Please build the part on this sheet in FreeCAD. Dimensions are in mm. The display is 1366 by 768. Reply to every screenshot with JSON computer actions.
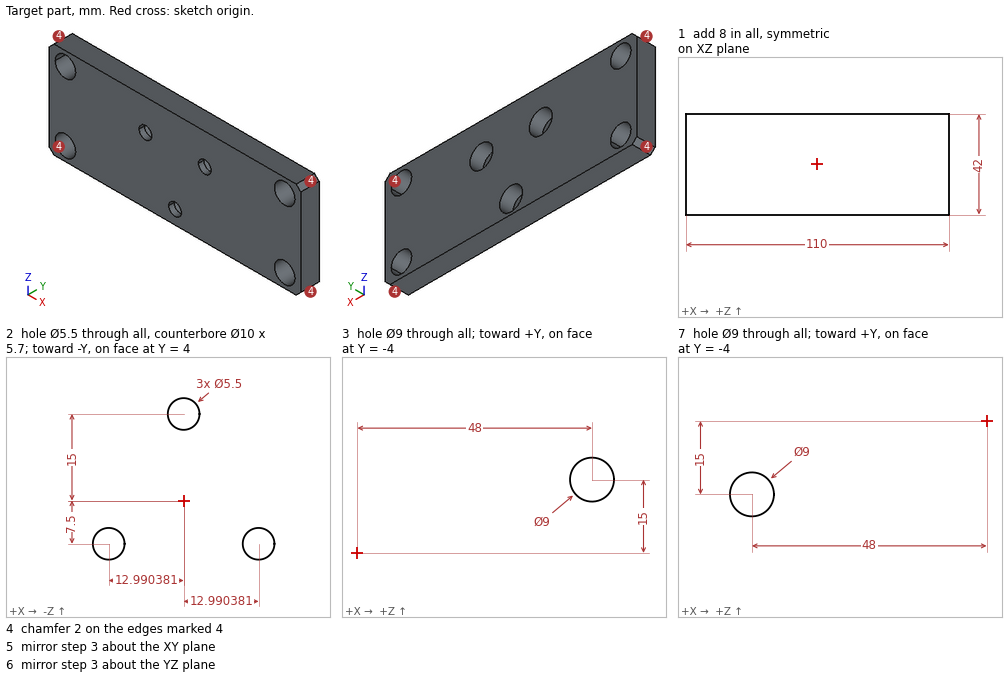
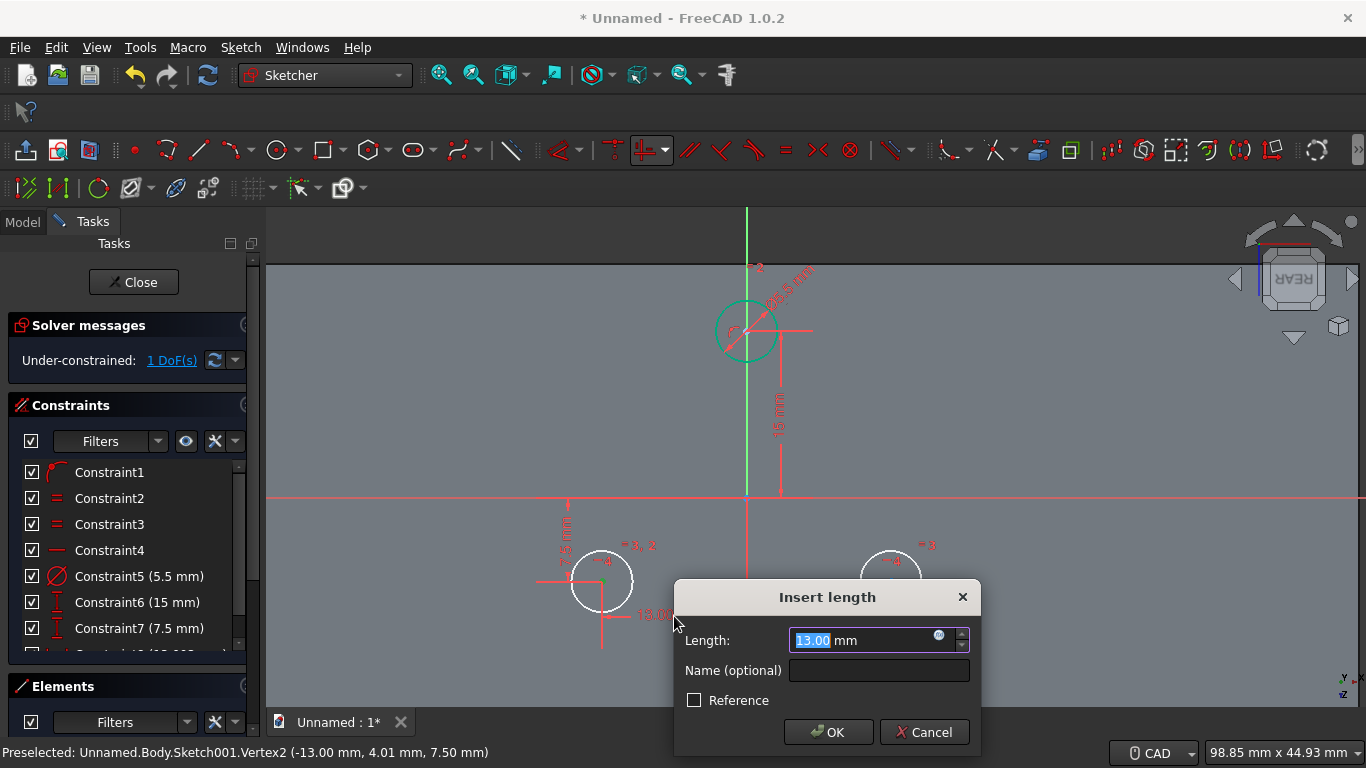
{"action": "type", "text": "12.990381"}
{"action": "key", "text": "Return"}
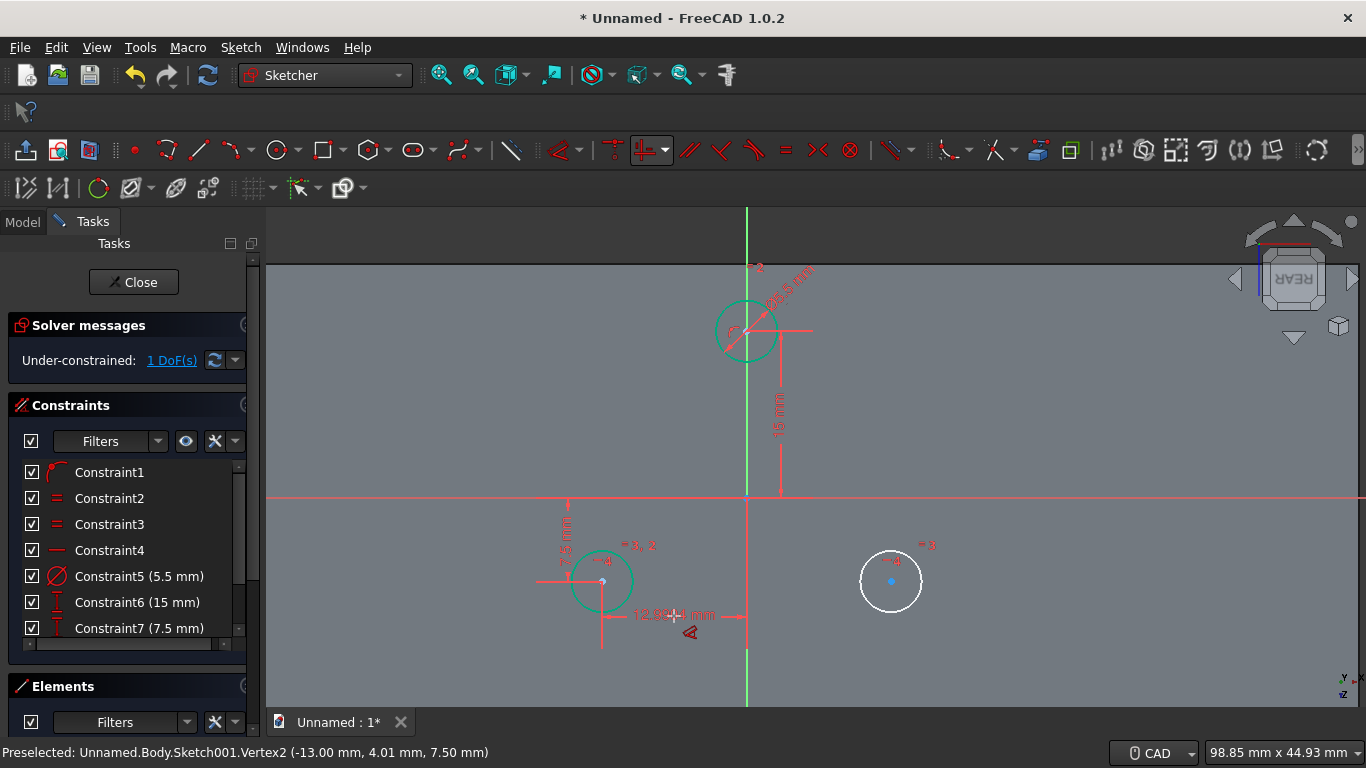
{"action": "left_click", "coordinate": [891, 582]}
{"action": "left_click", "coordinate": [819, 616]}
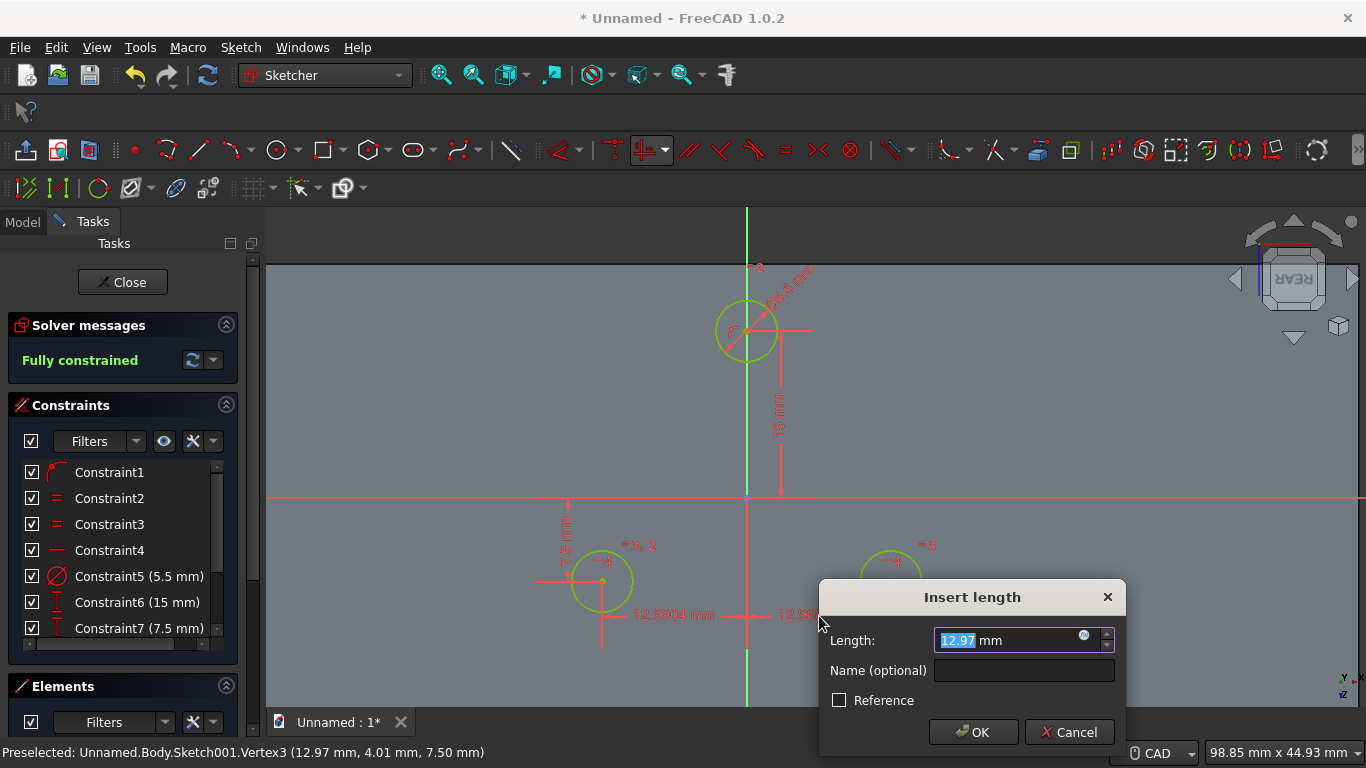
{"action": "type", "text": "12.990381"}
{"action": "key", "text": "Return"}
{"action": "key", "text": "Escape"}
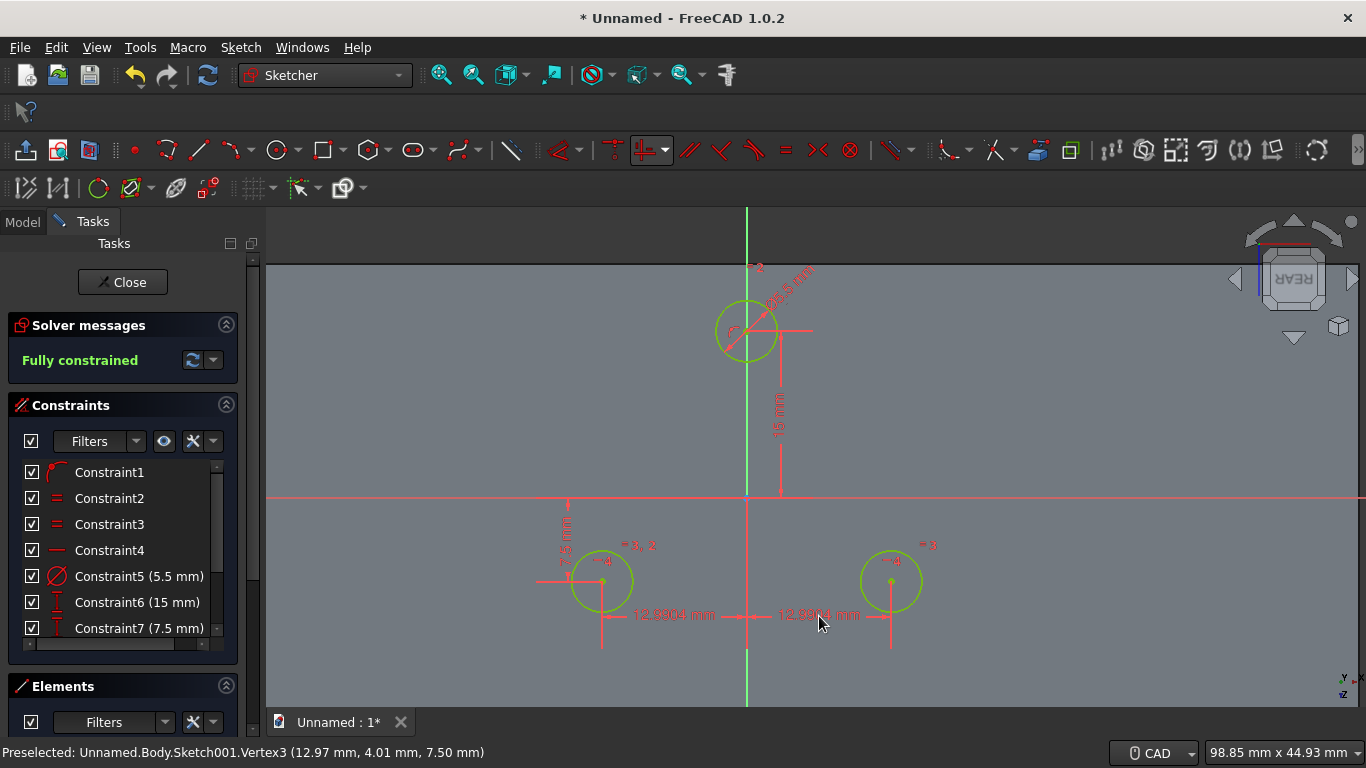
{"action": "left_click", "coordinate": [123, 282]}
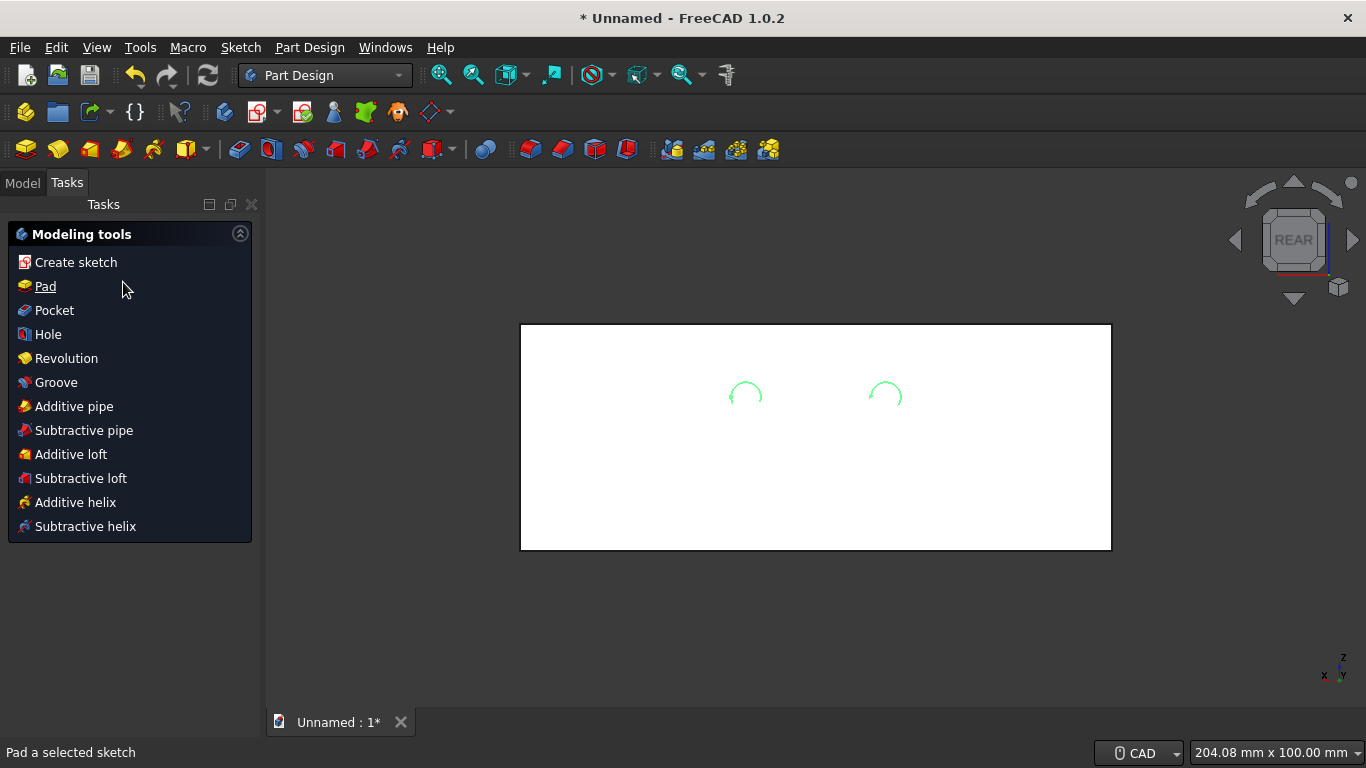
{"action": "left_click", "coordinate": [272, 150]}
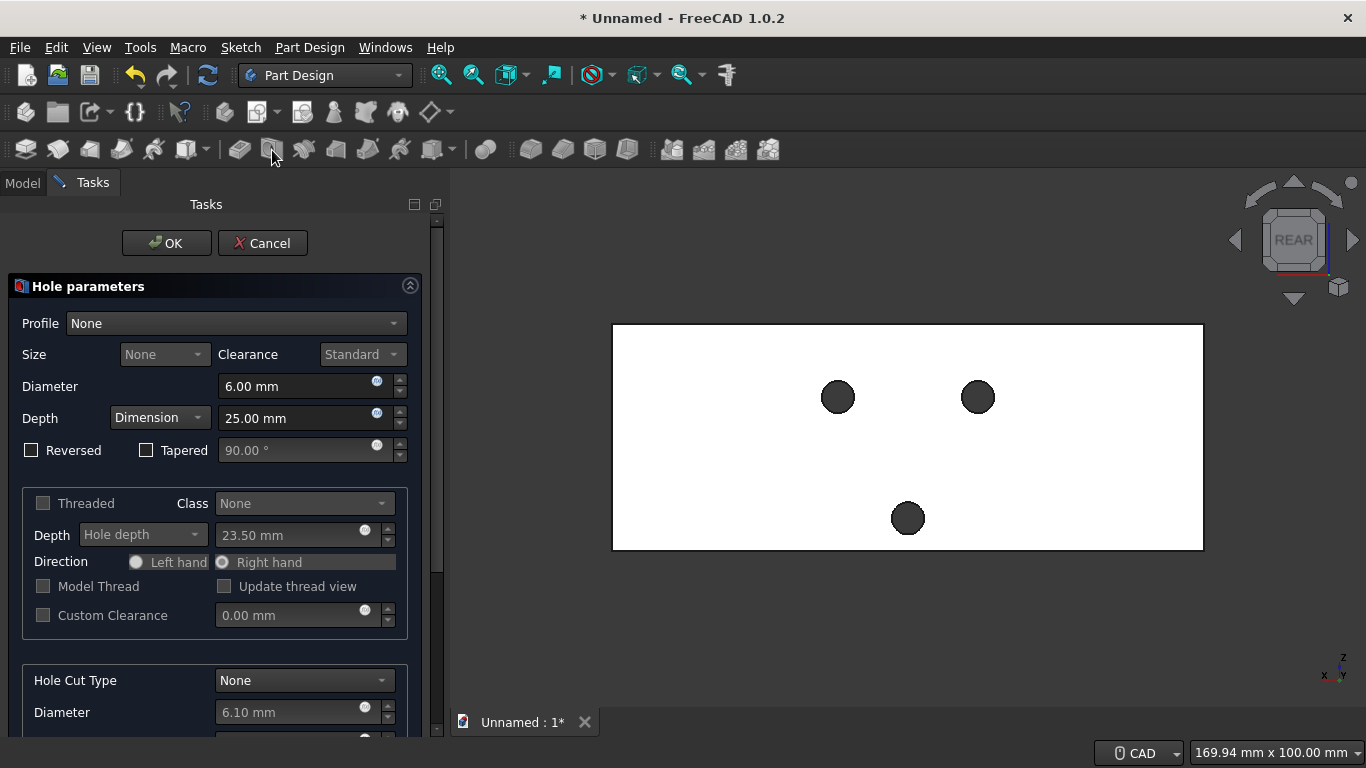
{"action": "triple_click", "coordinate": [305, 386]}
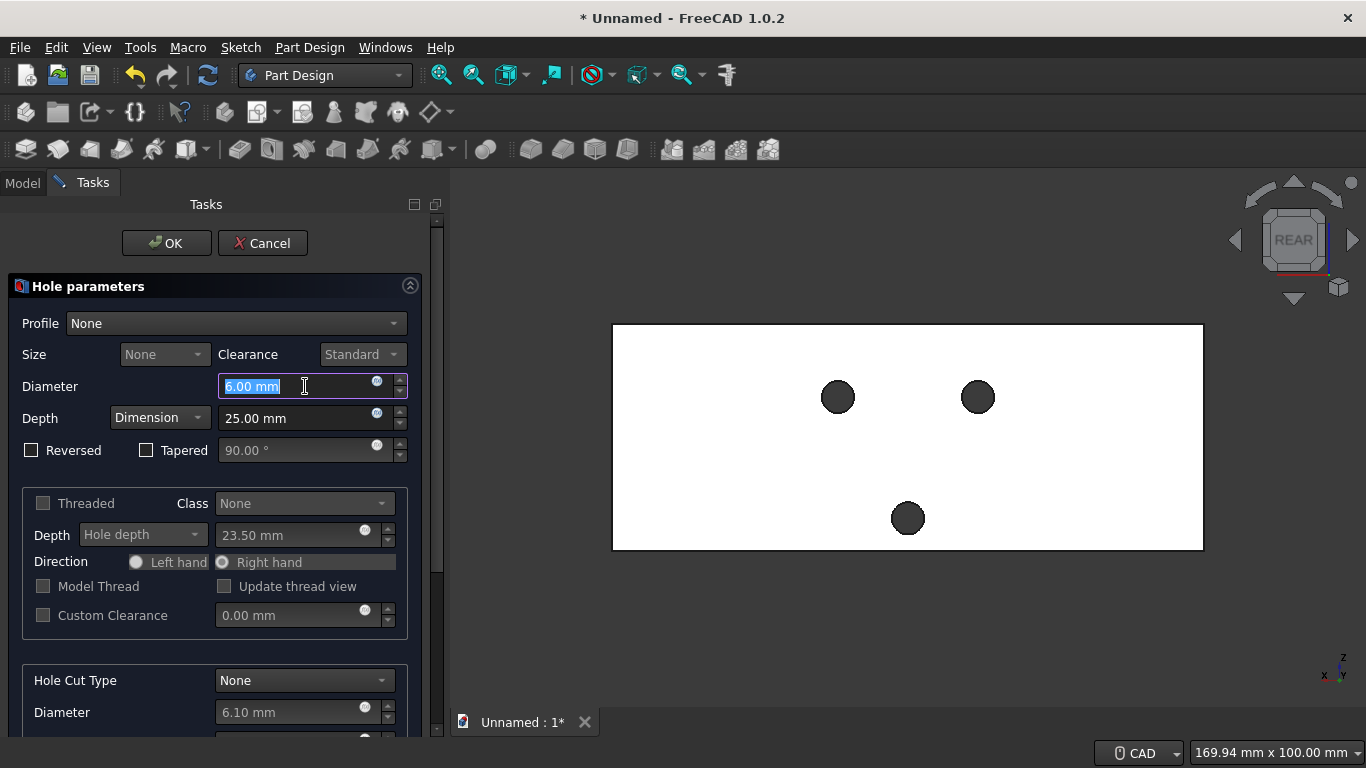
{"action": "type", "text": "5.5"}
{"action": "key", "text": "Tab"}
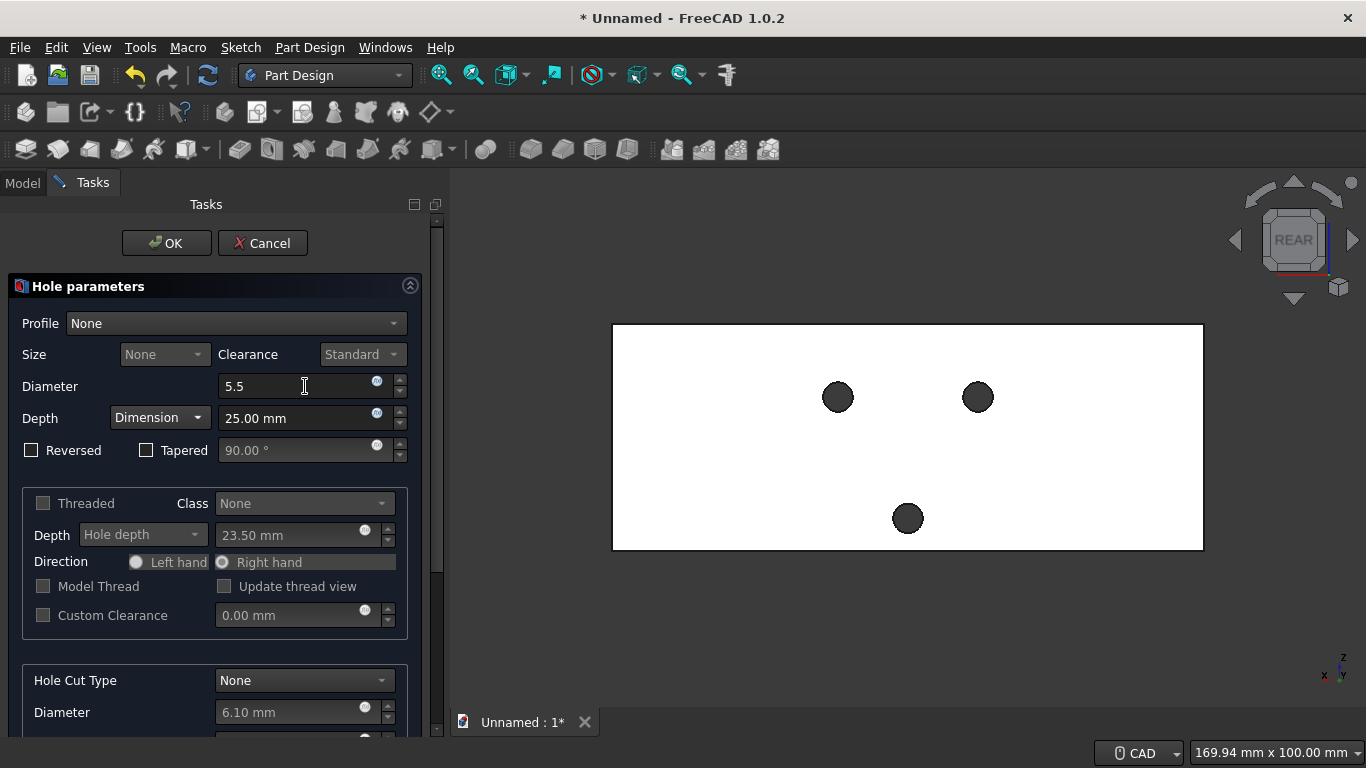
{"action": "left_click", "coordinate": [161, 418]}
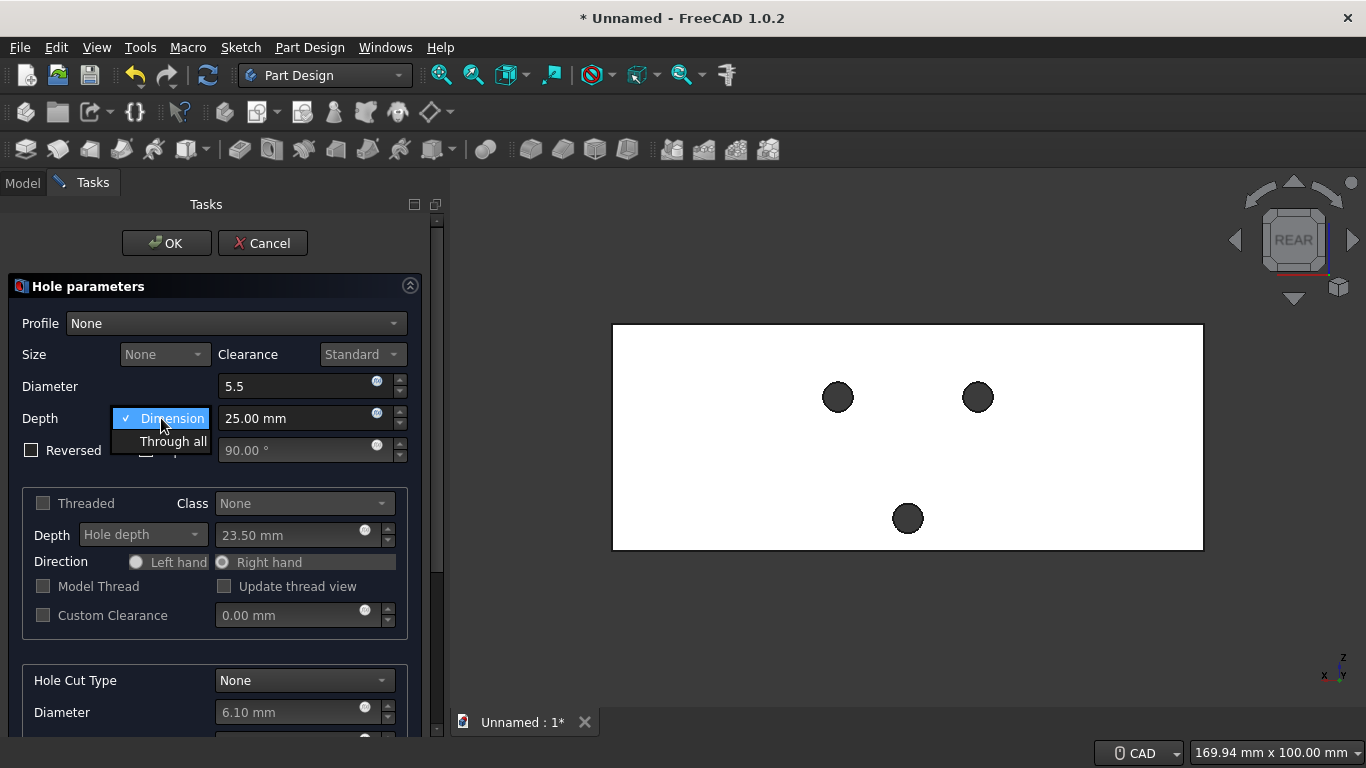
{"action": "left_click", "coordinate": [160, 442]}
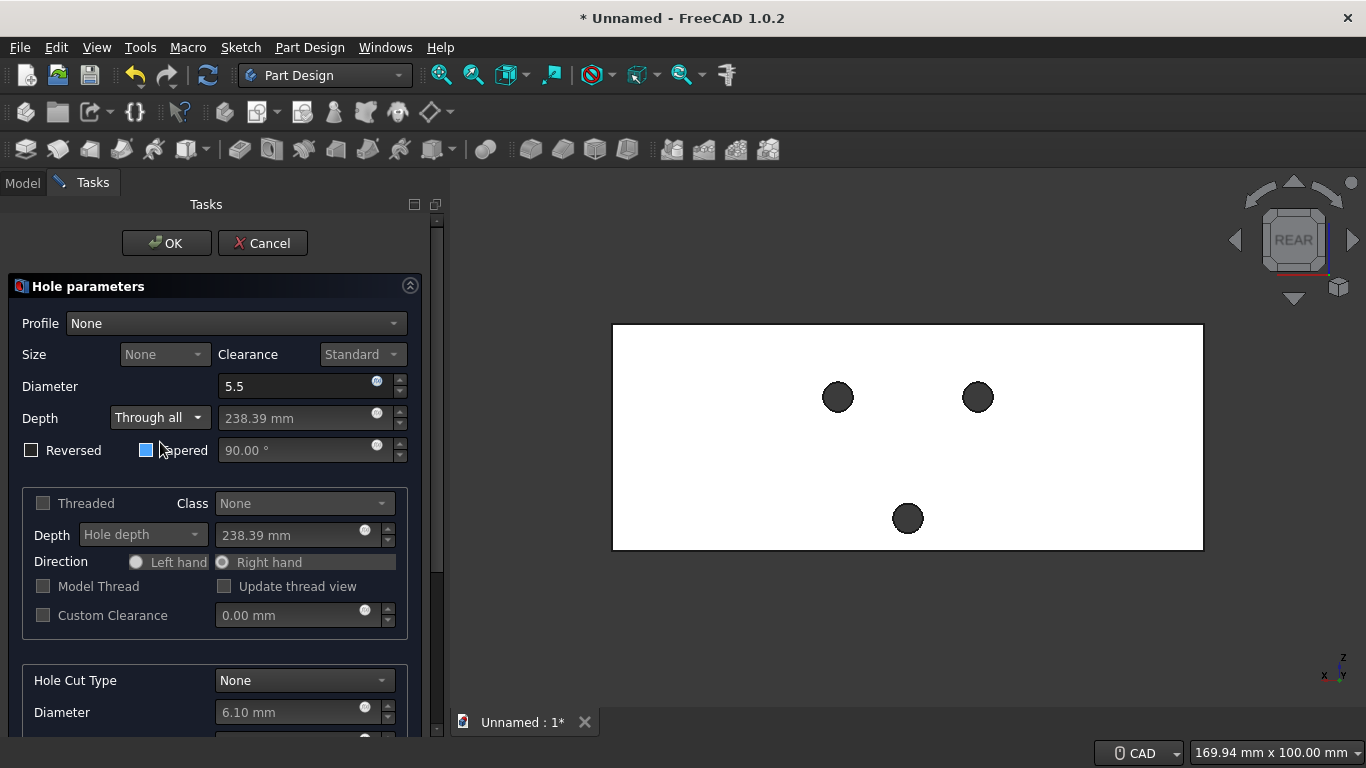
{"action": "left_click", "coordinate": [306, 680]}